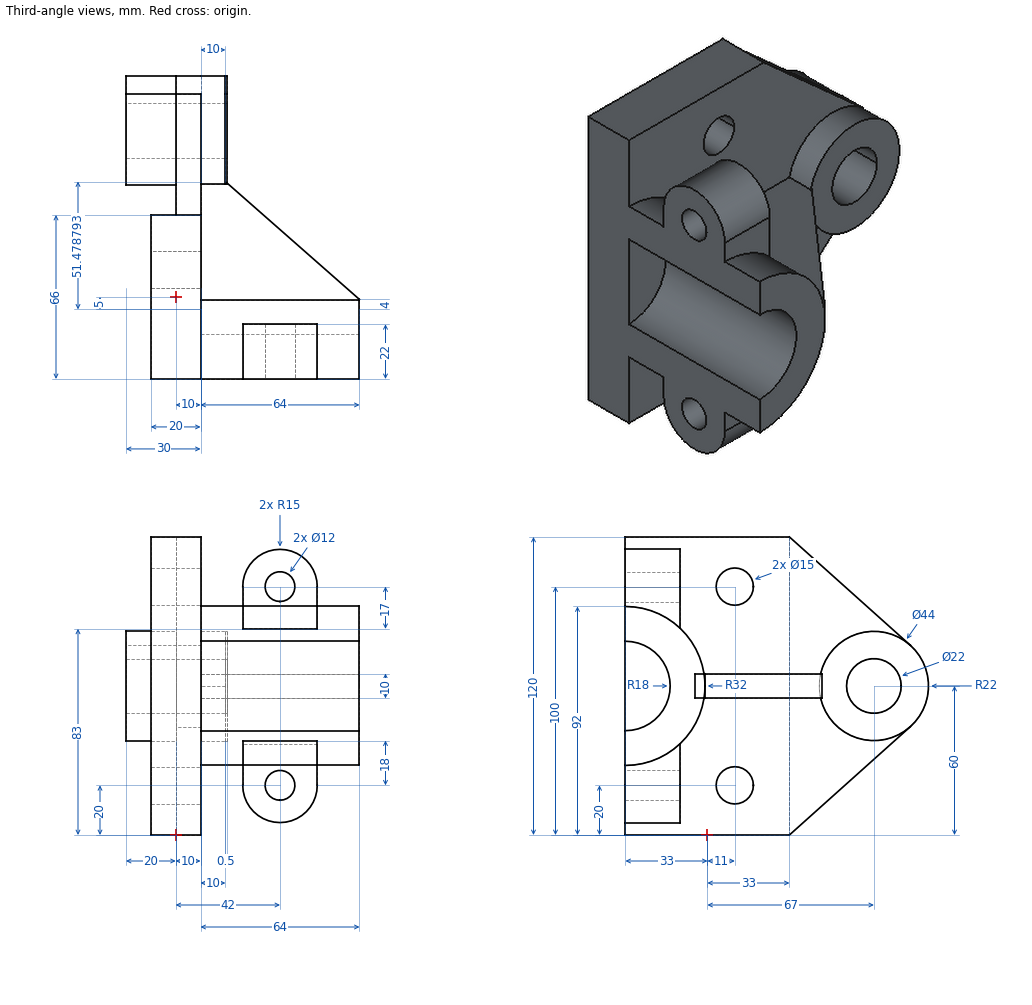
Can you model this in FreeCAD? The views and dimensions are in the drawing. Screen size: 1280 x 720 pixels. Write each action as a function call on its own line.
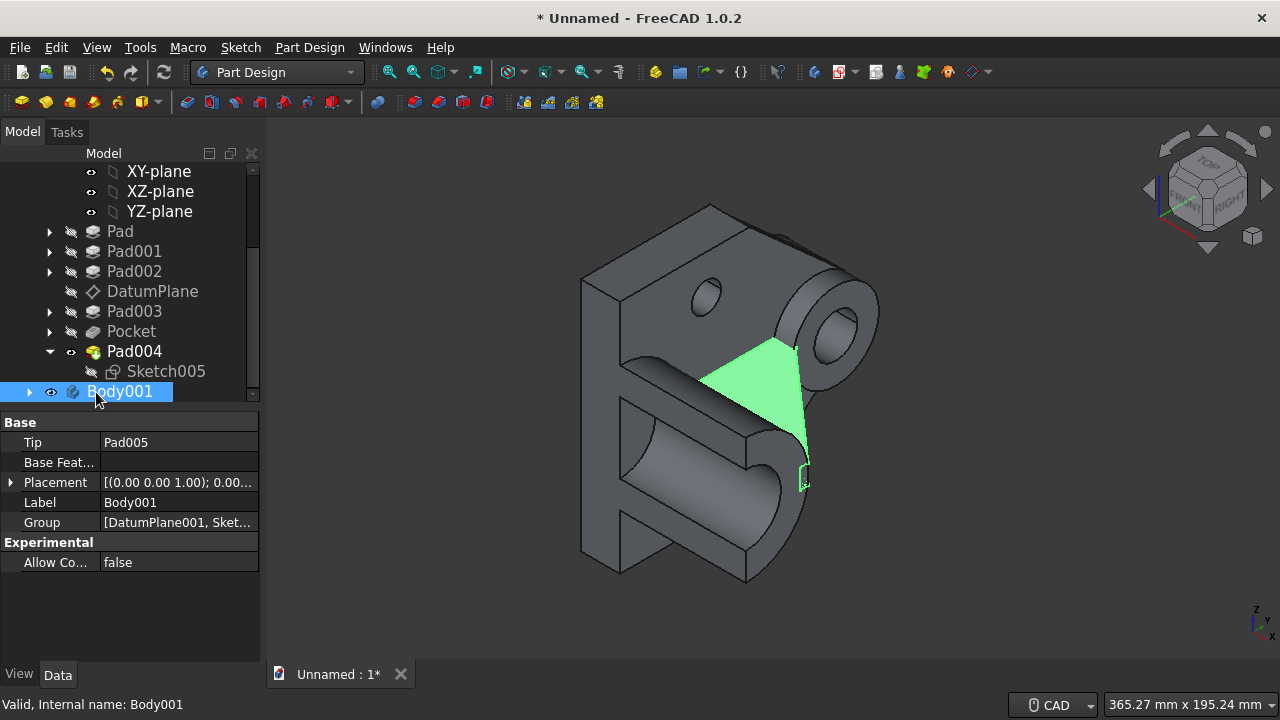
click(378, 102)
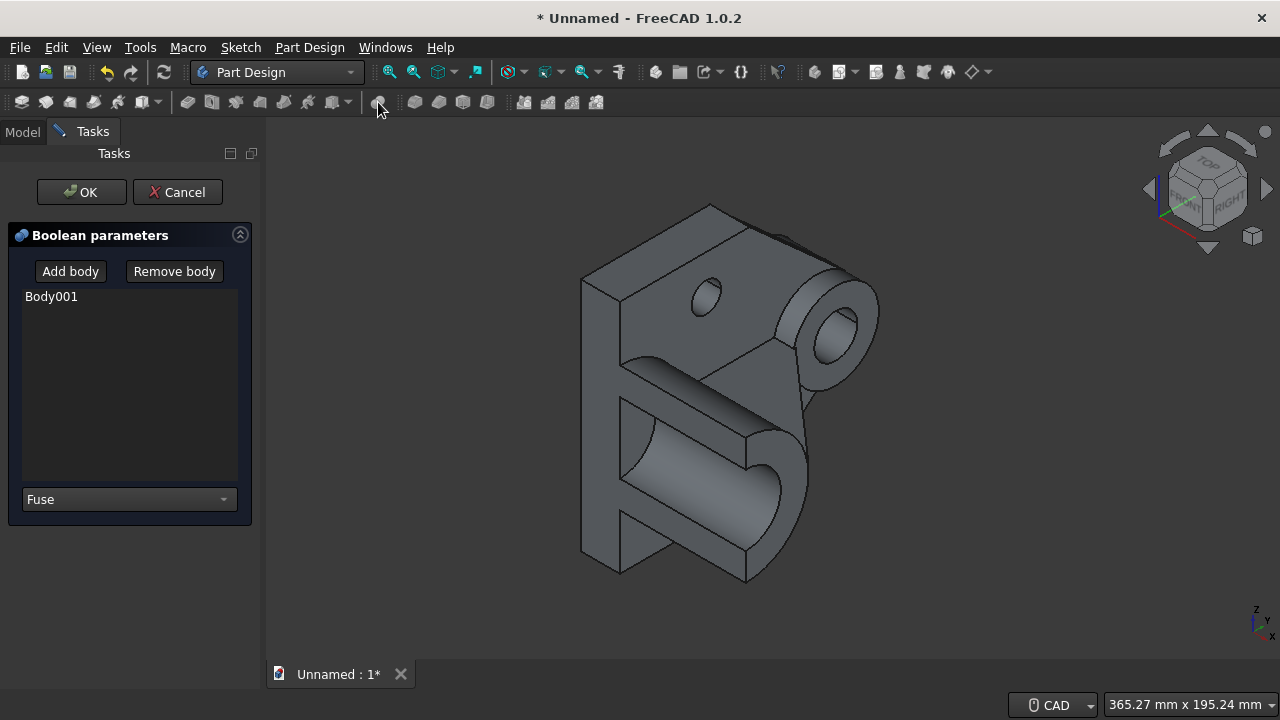
click(82, 192)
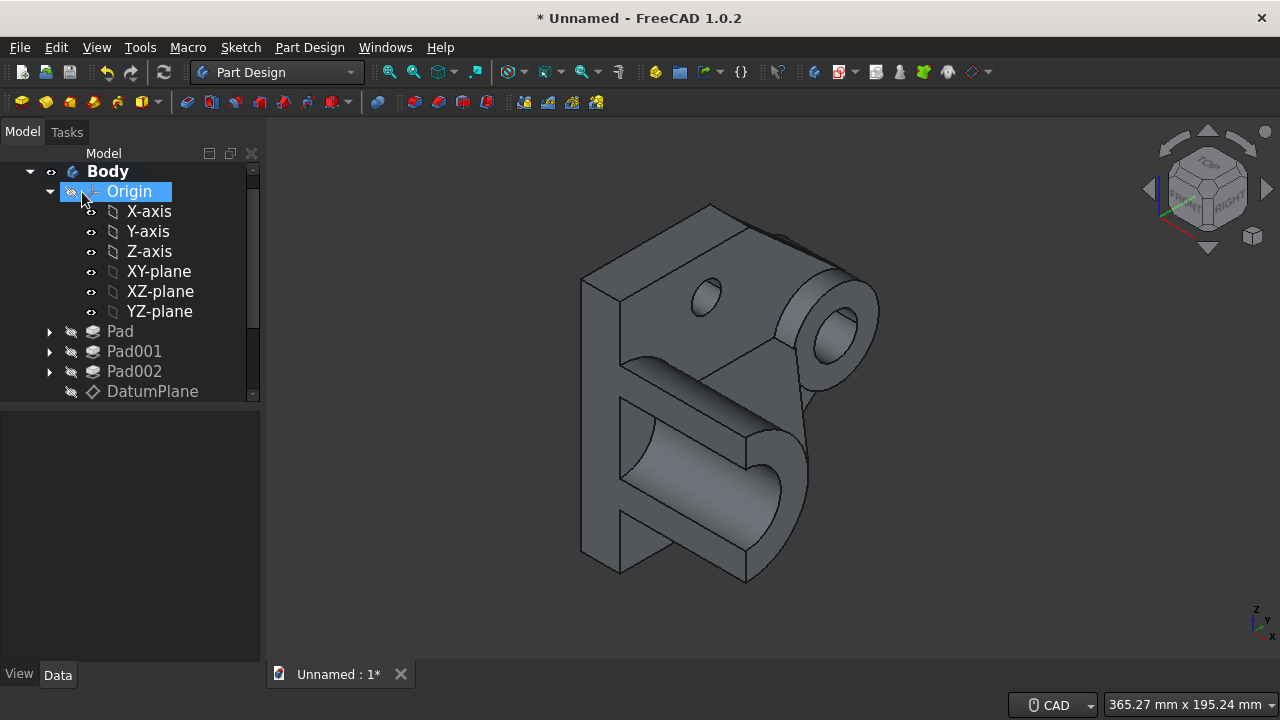
click(136, 312)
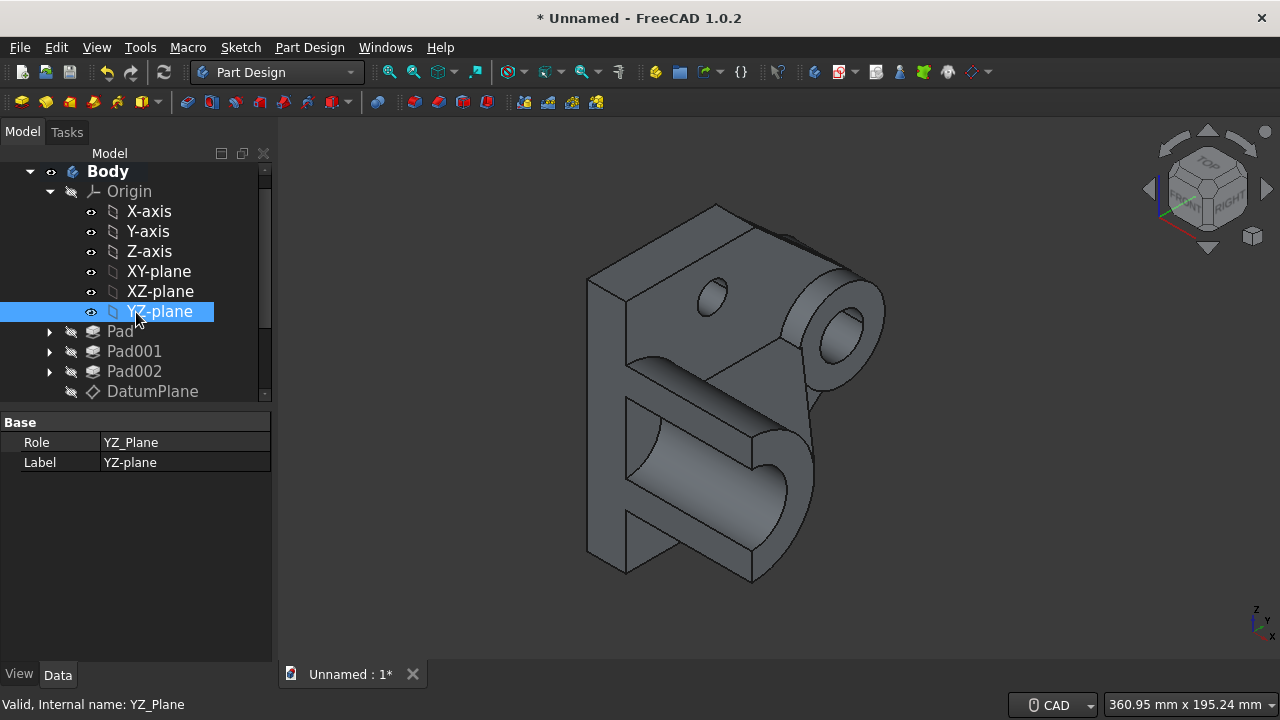
click(972, 72)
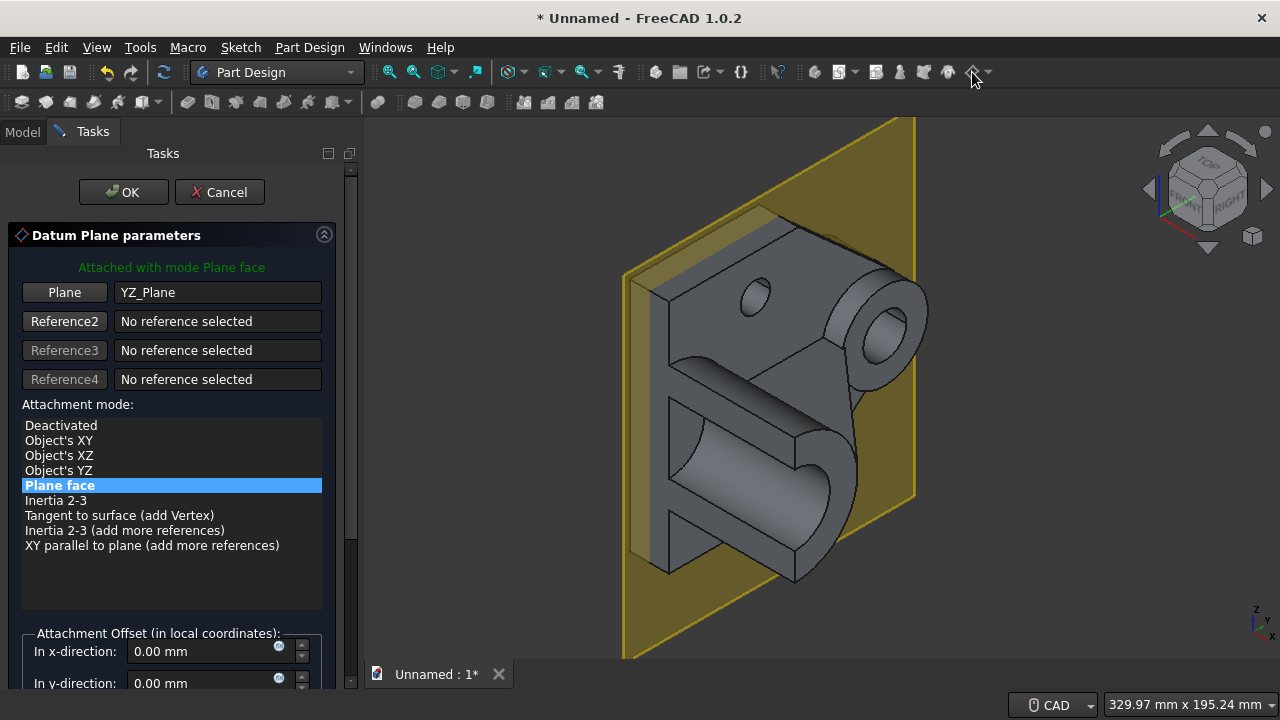
scroll(351, 426, down, 2)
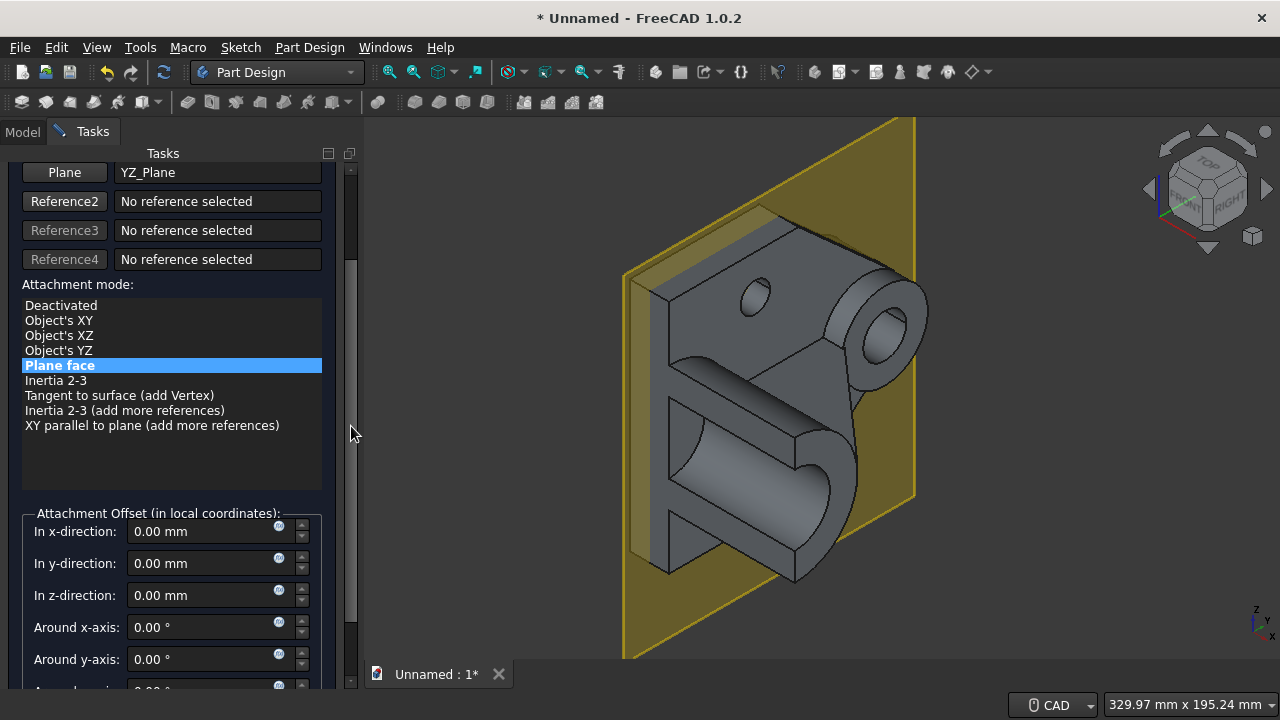
triple_click(210, 595)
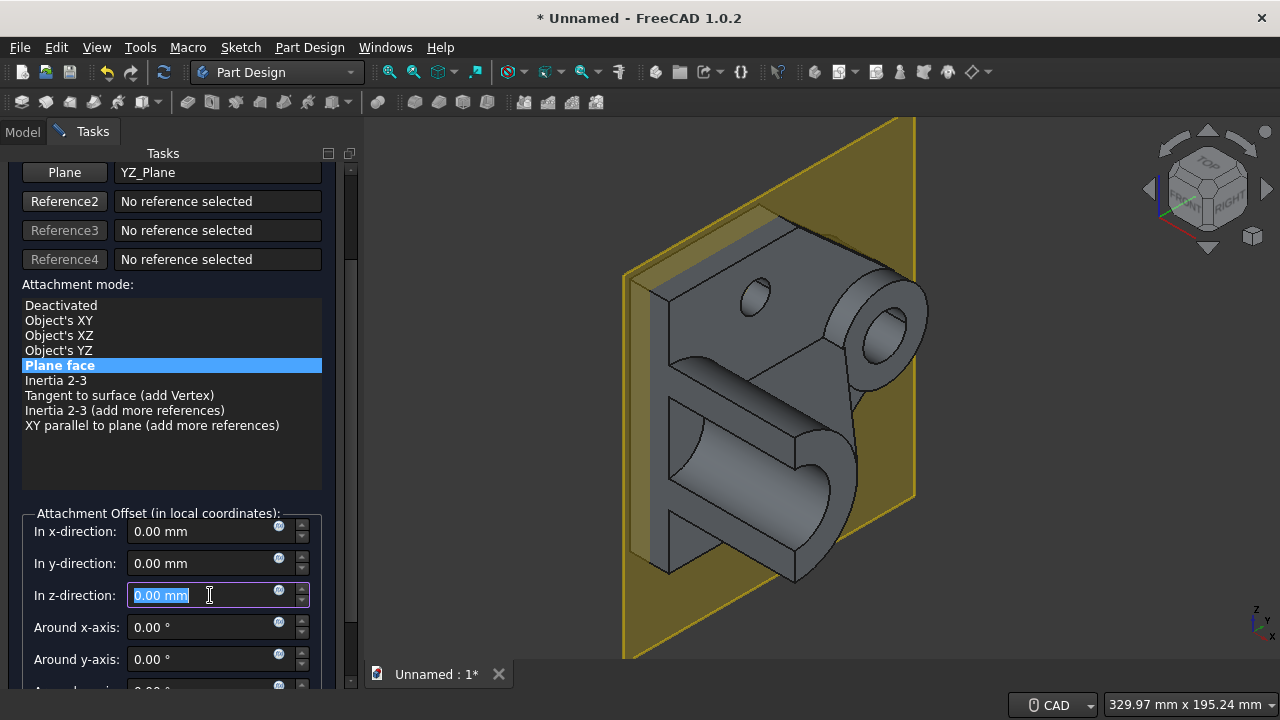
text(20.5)
key(Tab)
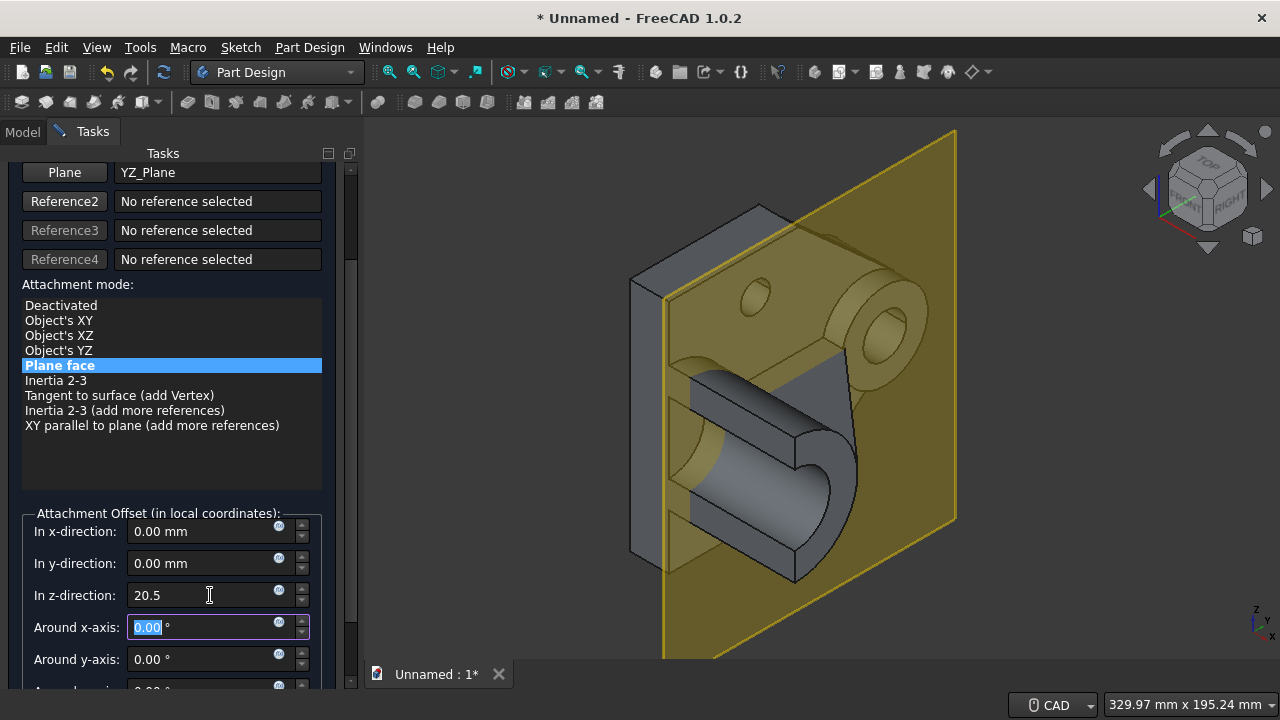
scroll(351, 426, up, 3)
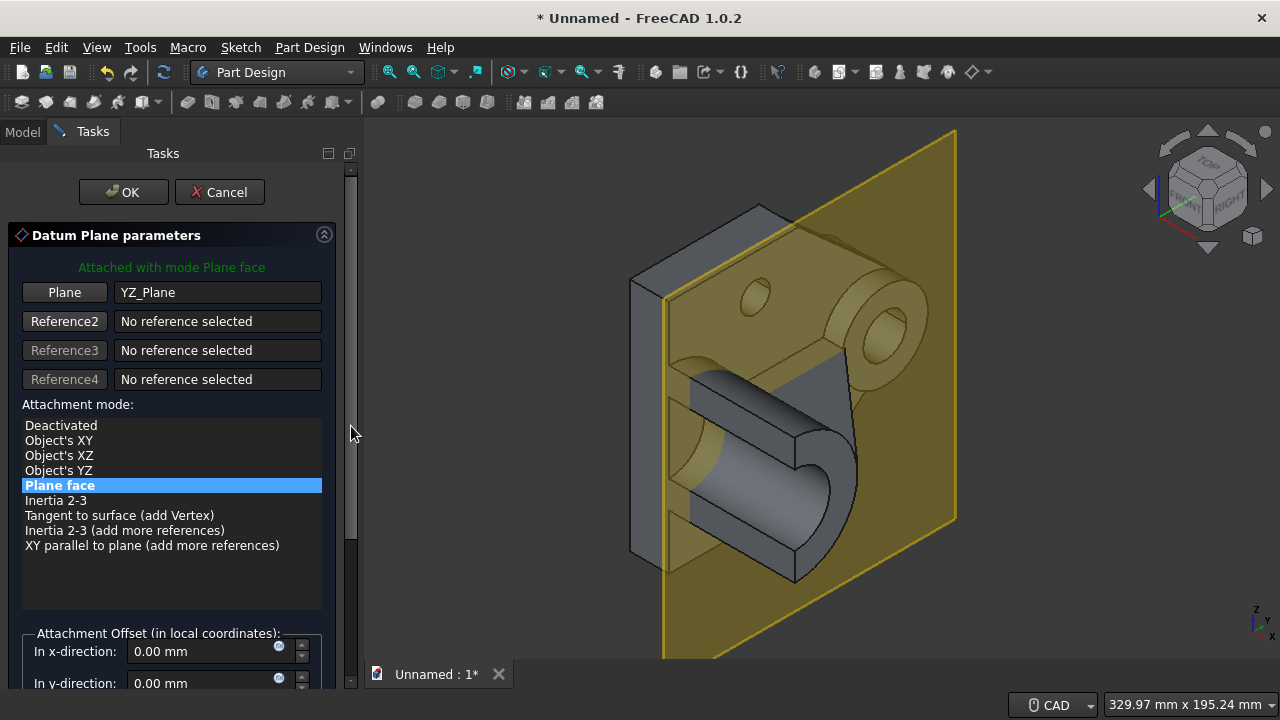
click(124, 192)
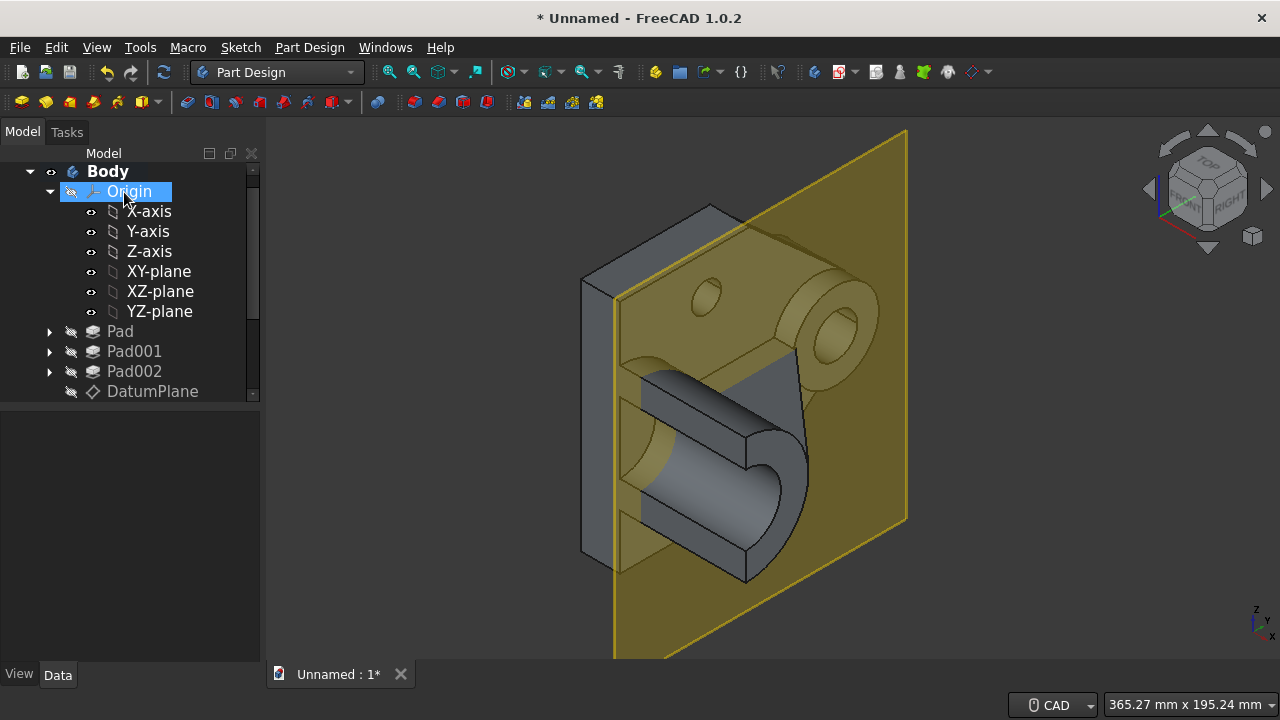
scroll(120, 287, down, 3)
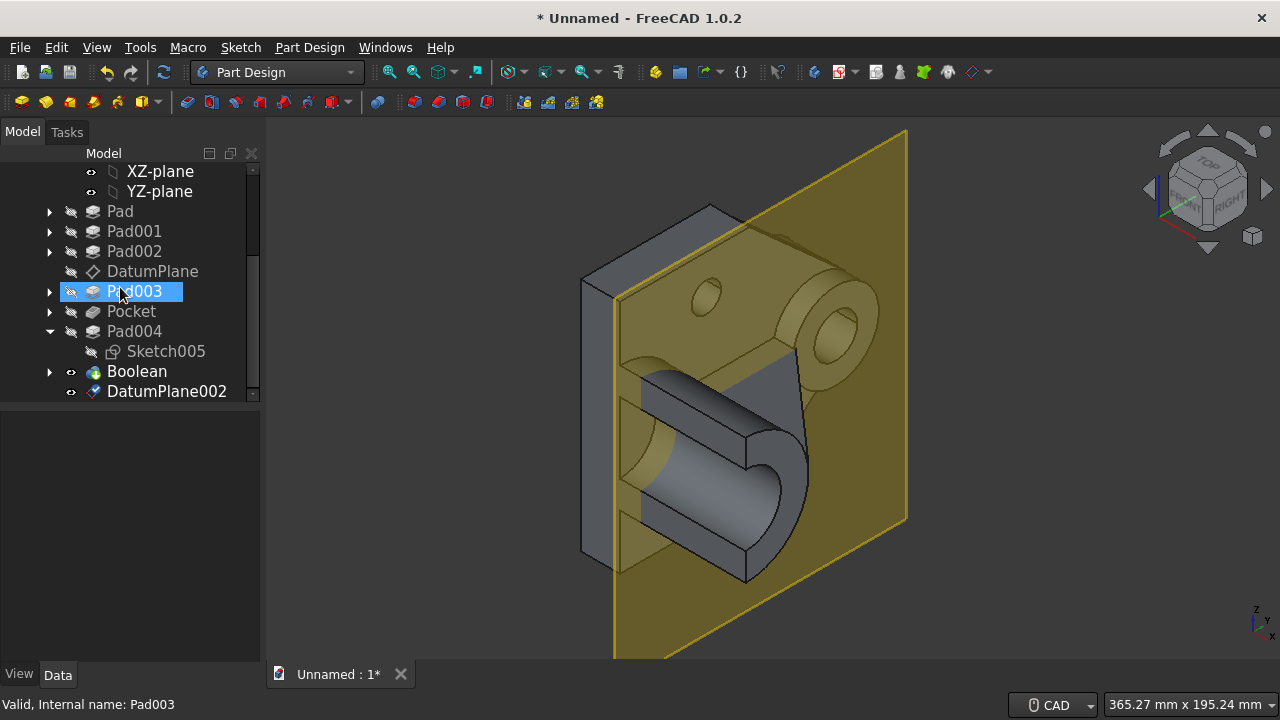
click(116, 392)